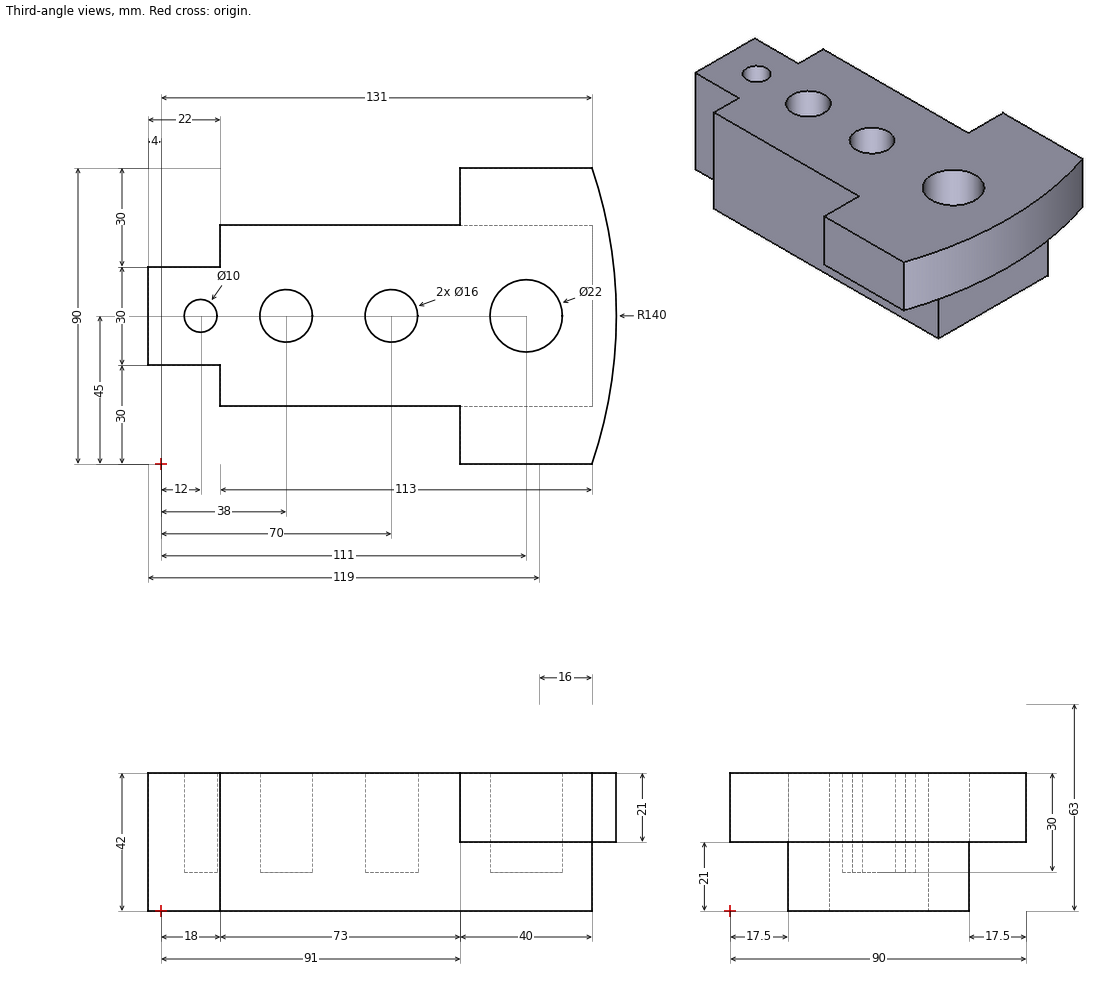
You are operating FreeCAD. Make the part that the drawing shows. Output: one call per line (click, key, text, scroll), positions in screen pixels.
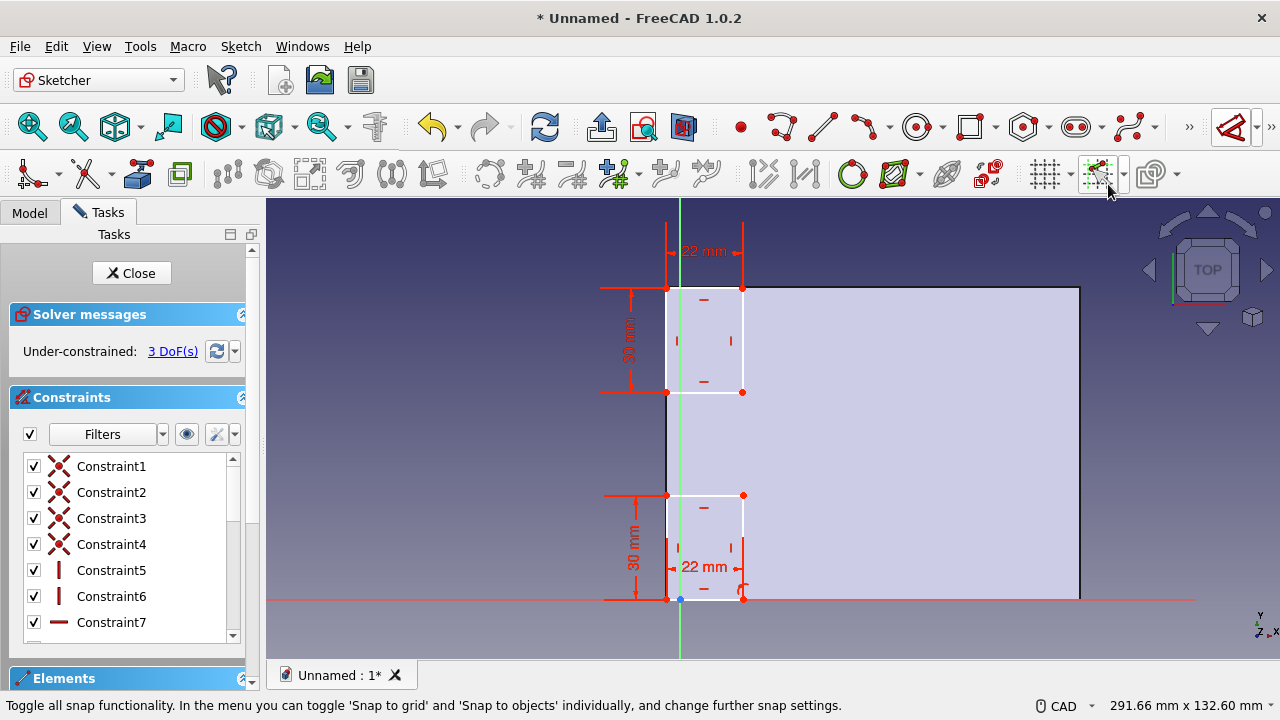
scroll(666, 288, up, 6)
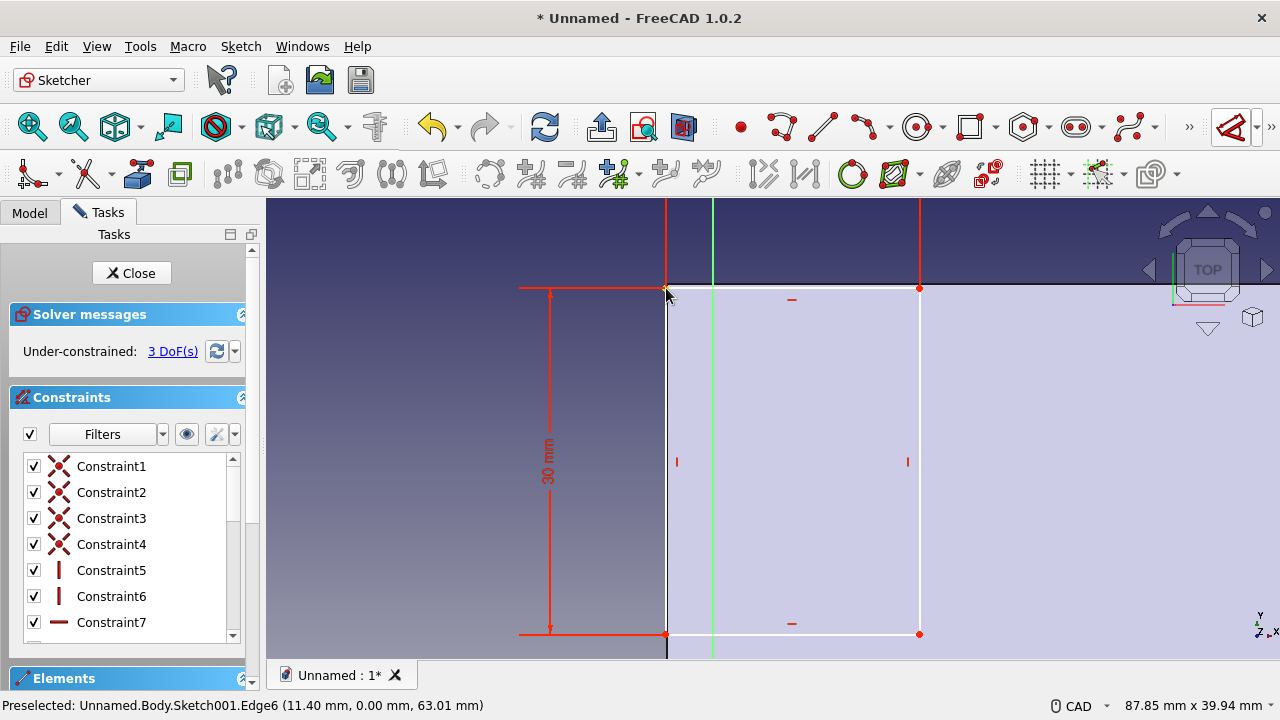
click(666, 288)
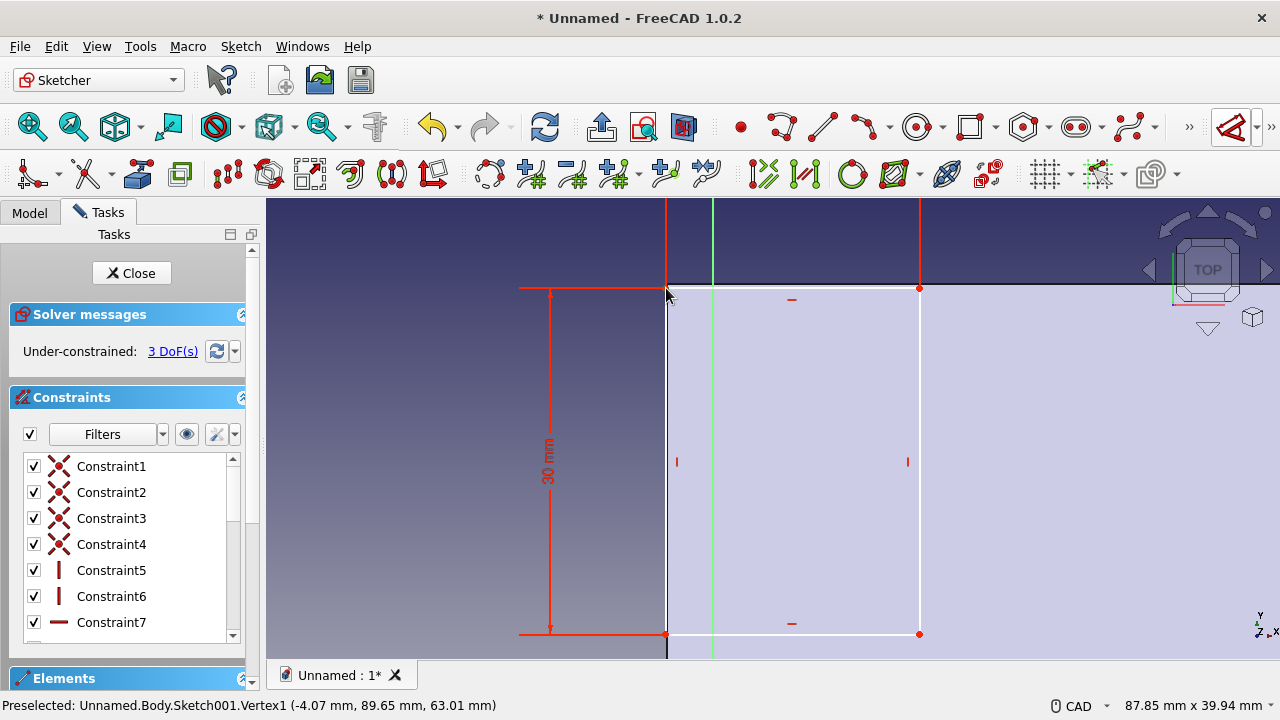
key(l)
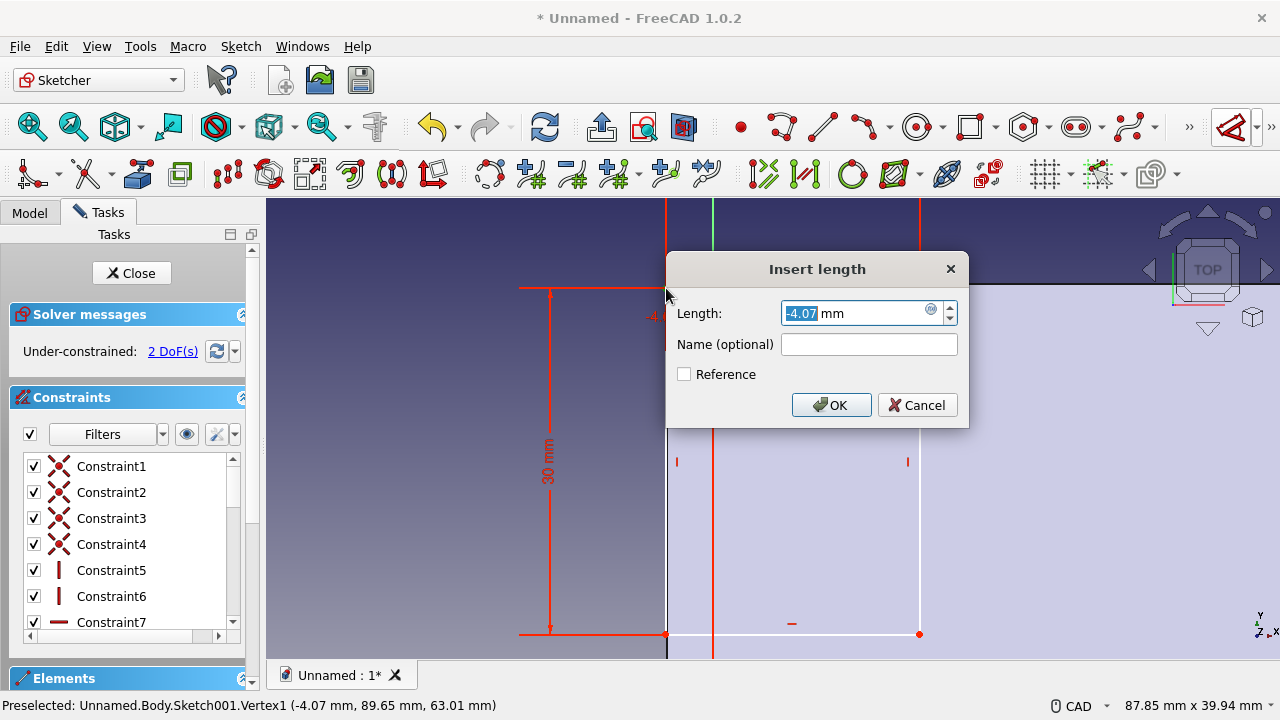
text(-4)
key(Return)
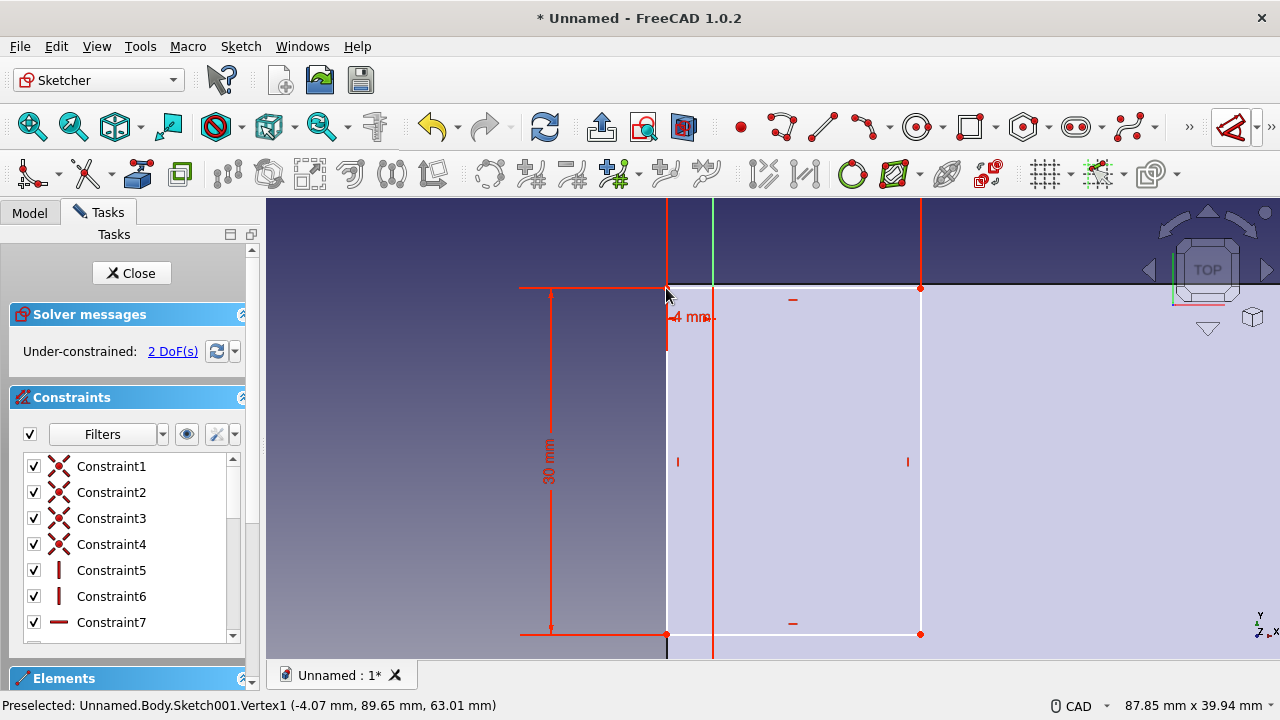
scroll(666, 267, down, 6)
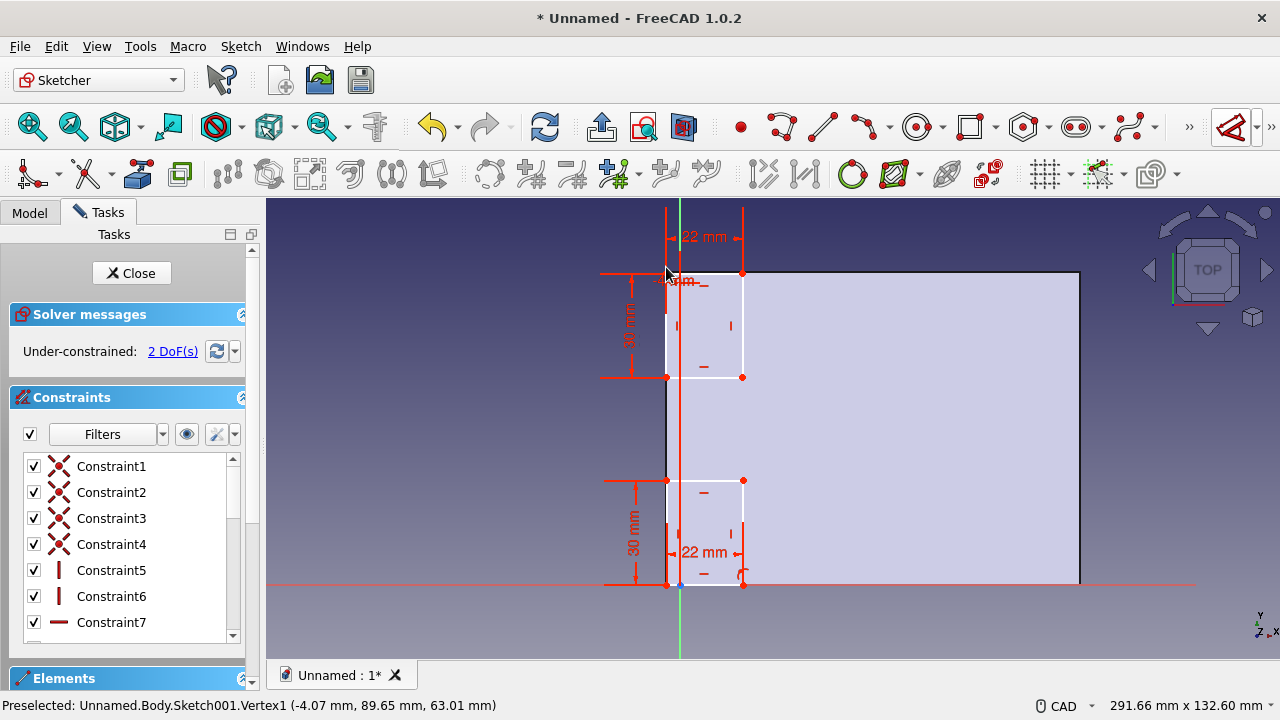
scroll(667, 481, up, 6)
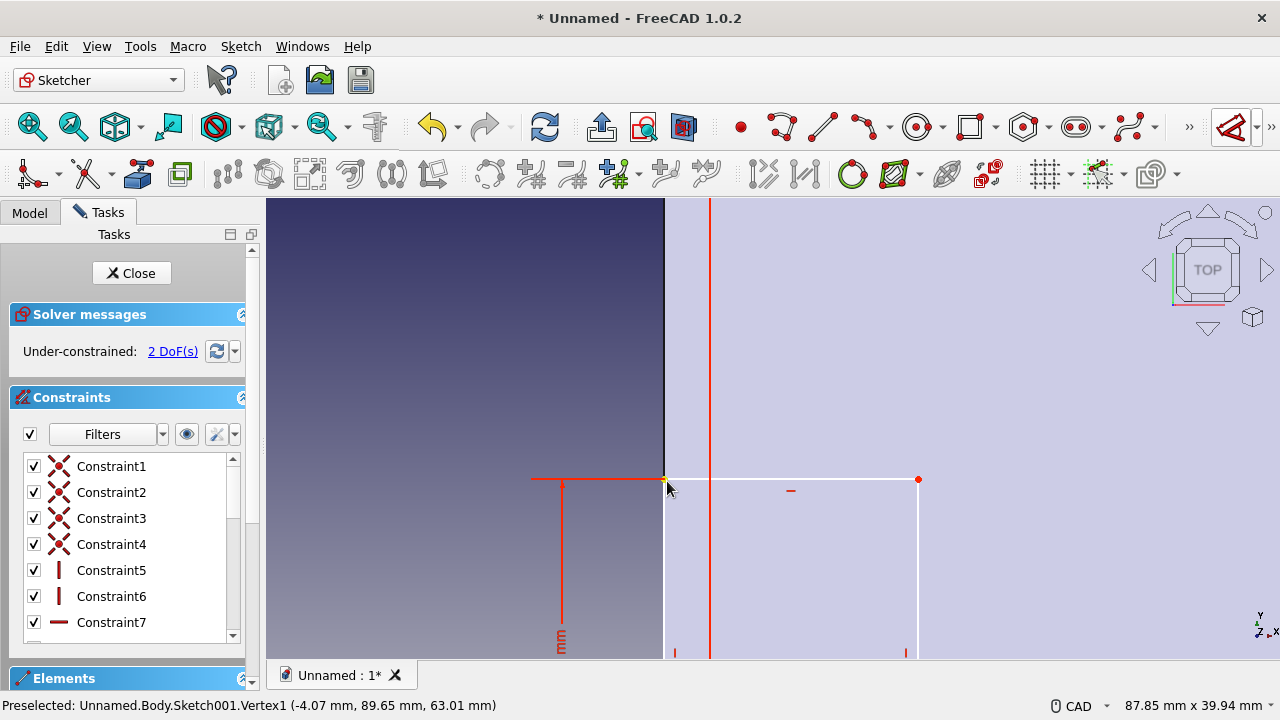
click(664, 479)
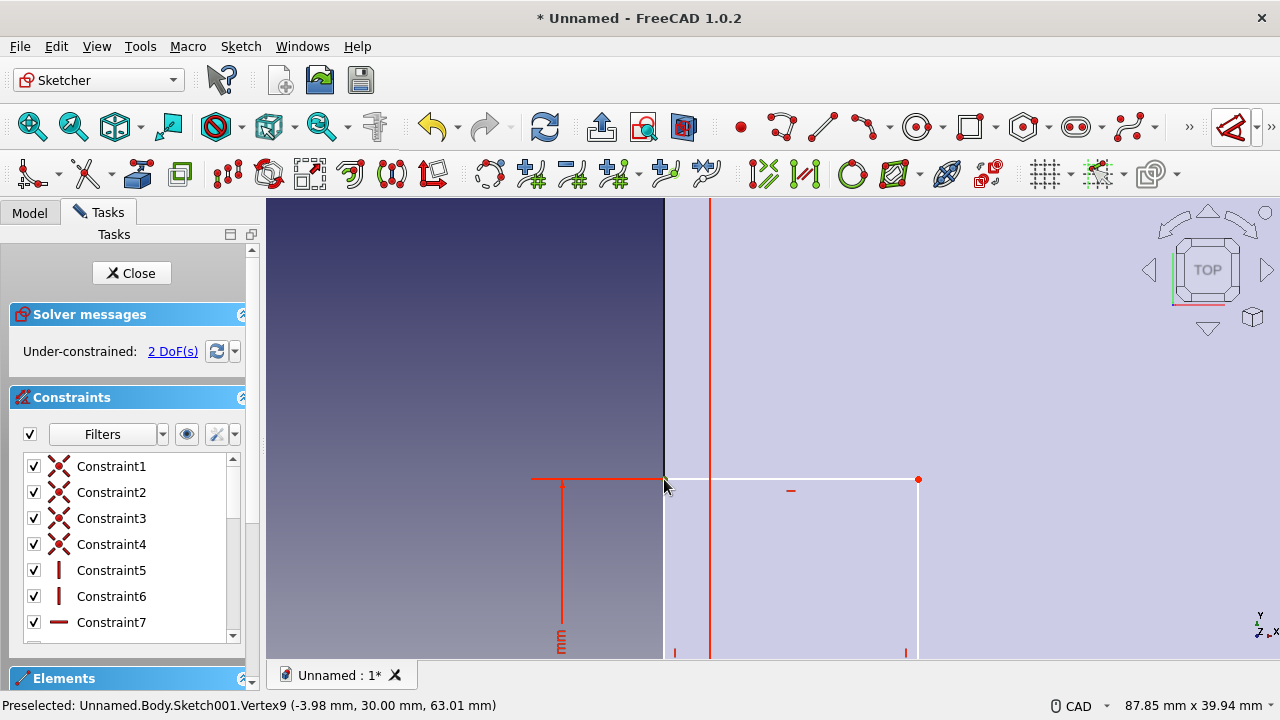
click(1256, 128)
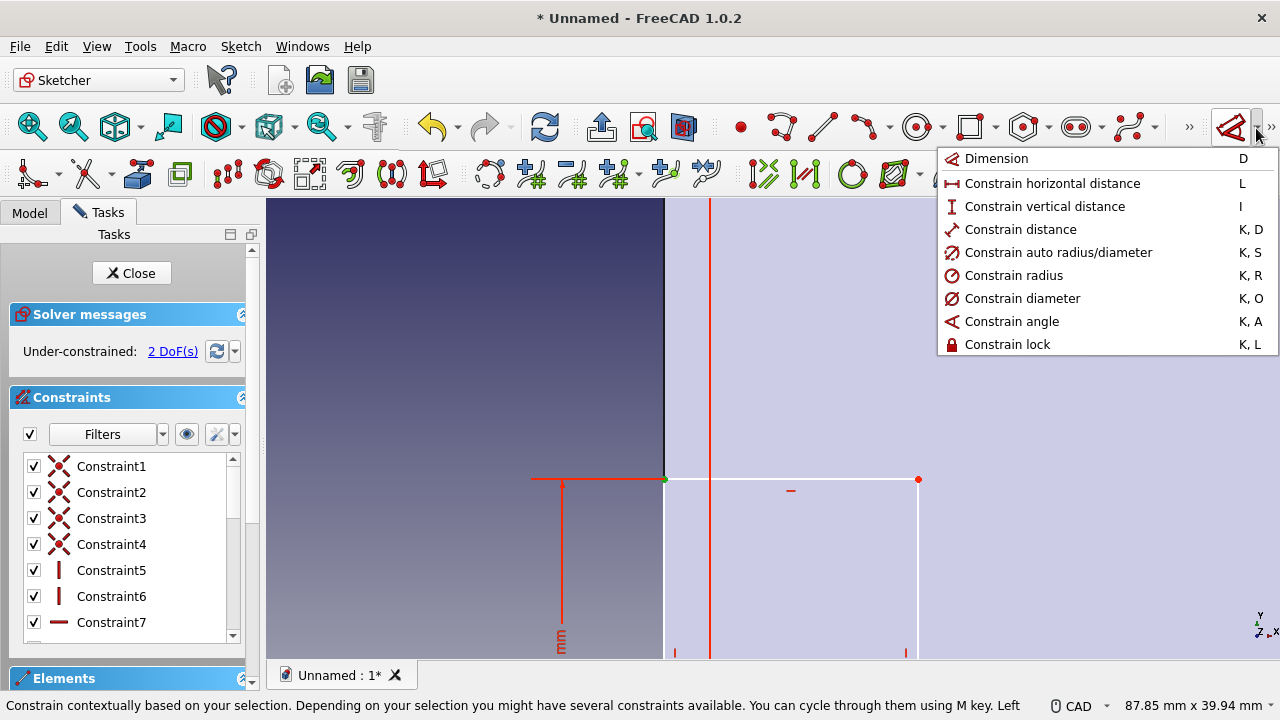
click(1108, 184)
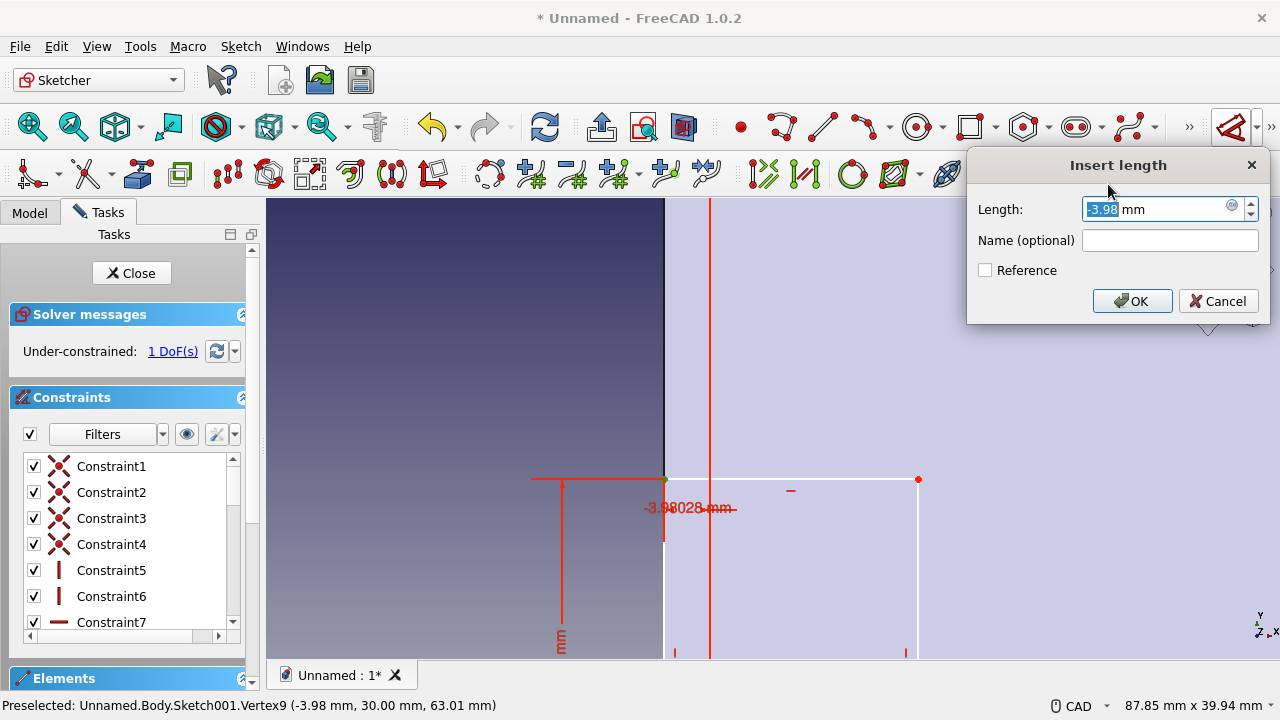
text(-4)
key(Return)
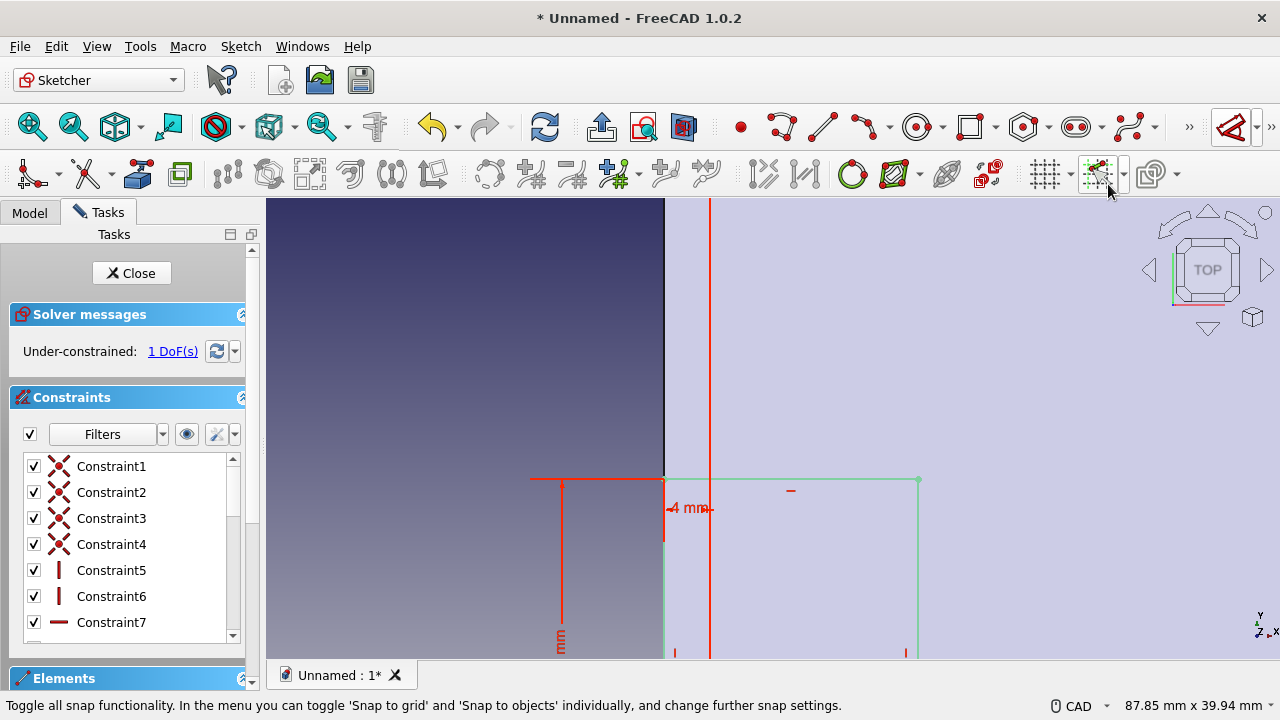
scroll(667, 481, down, 6)